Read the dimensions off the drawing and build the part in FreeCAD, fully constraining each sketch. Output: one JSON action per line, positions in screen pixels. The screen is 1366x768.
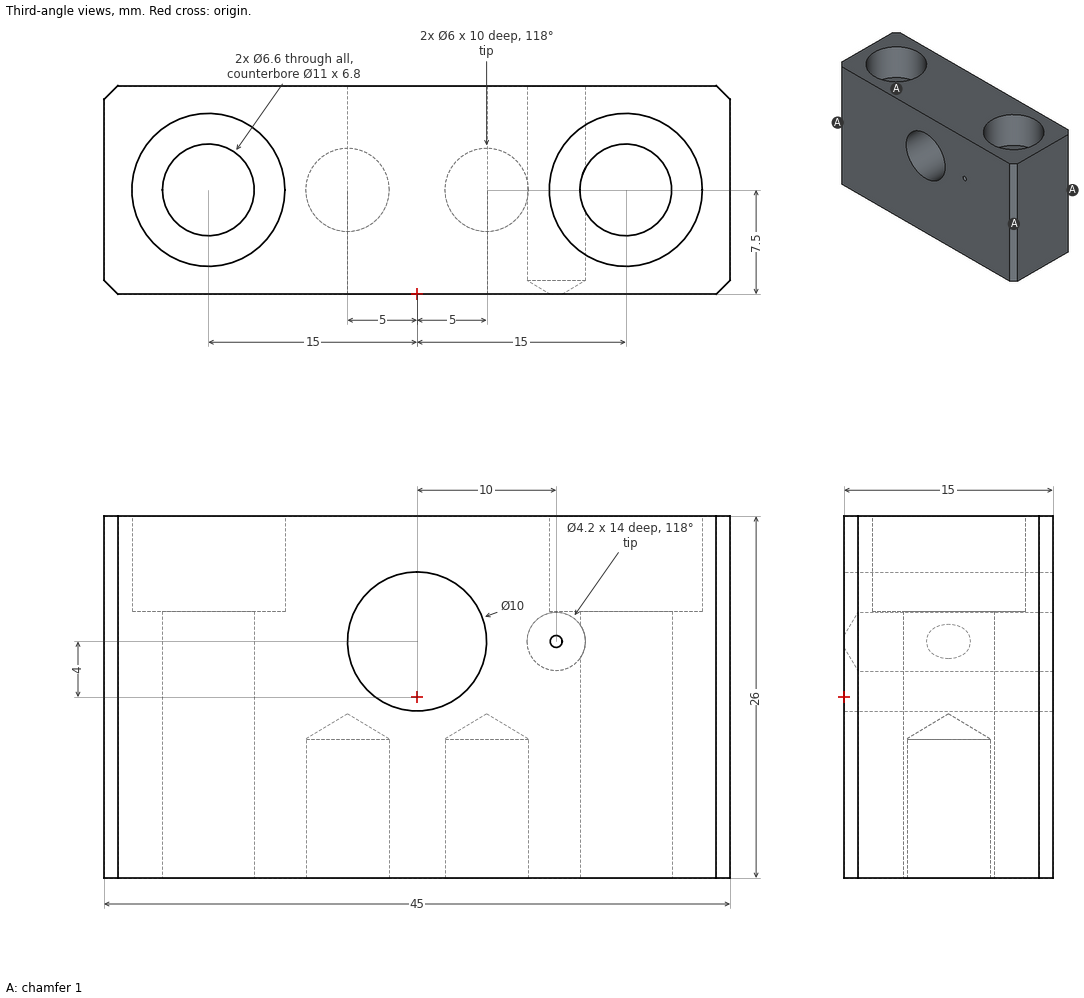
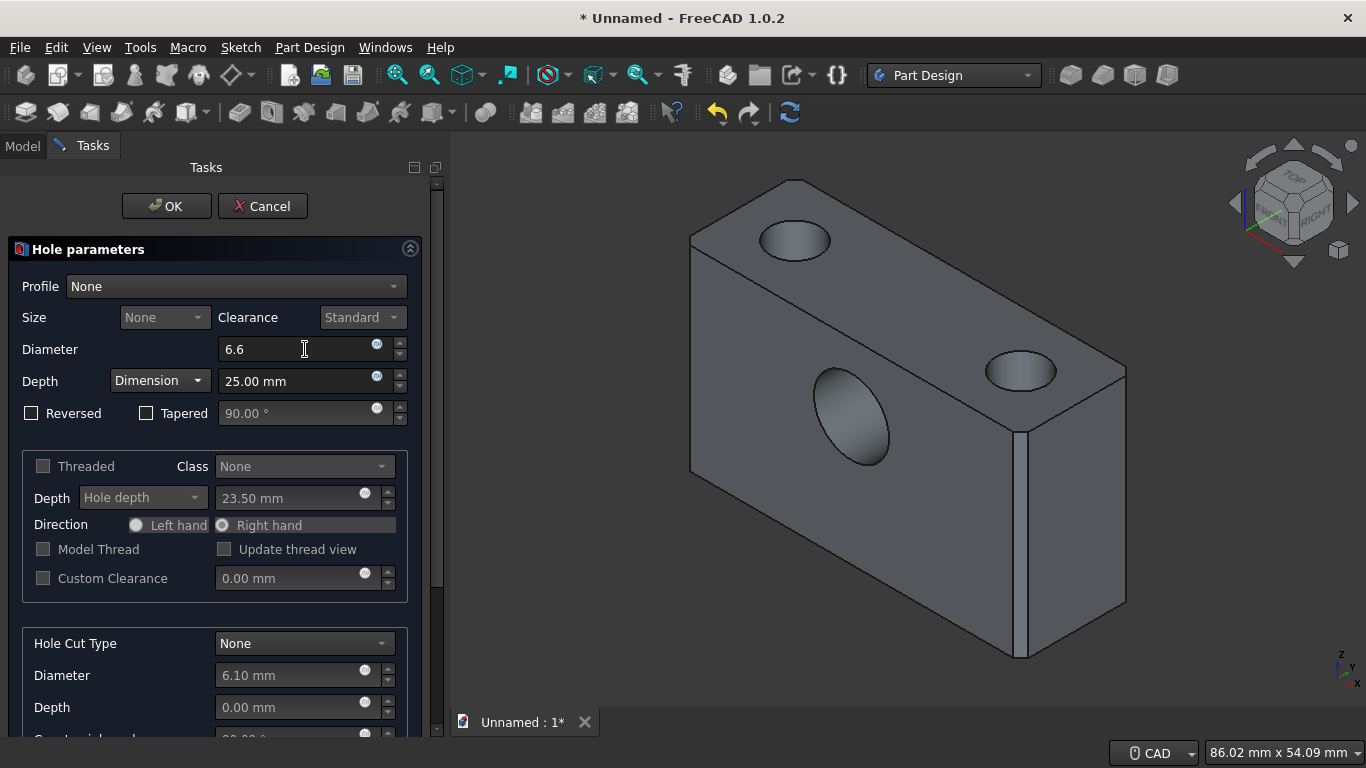
{"action": "left_click", "coordinate": [161, 380]}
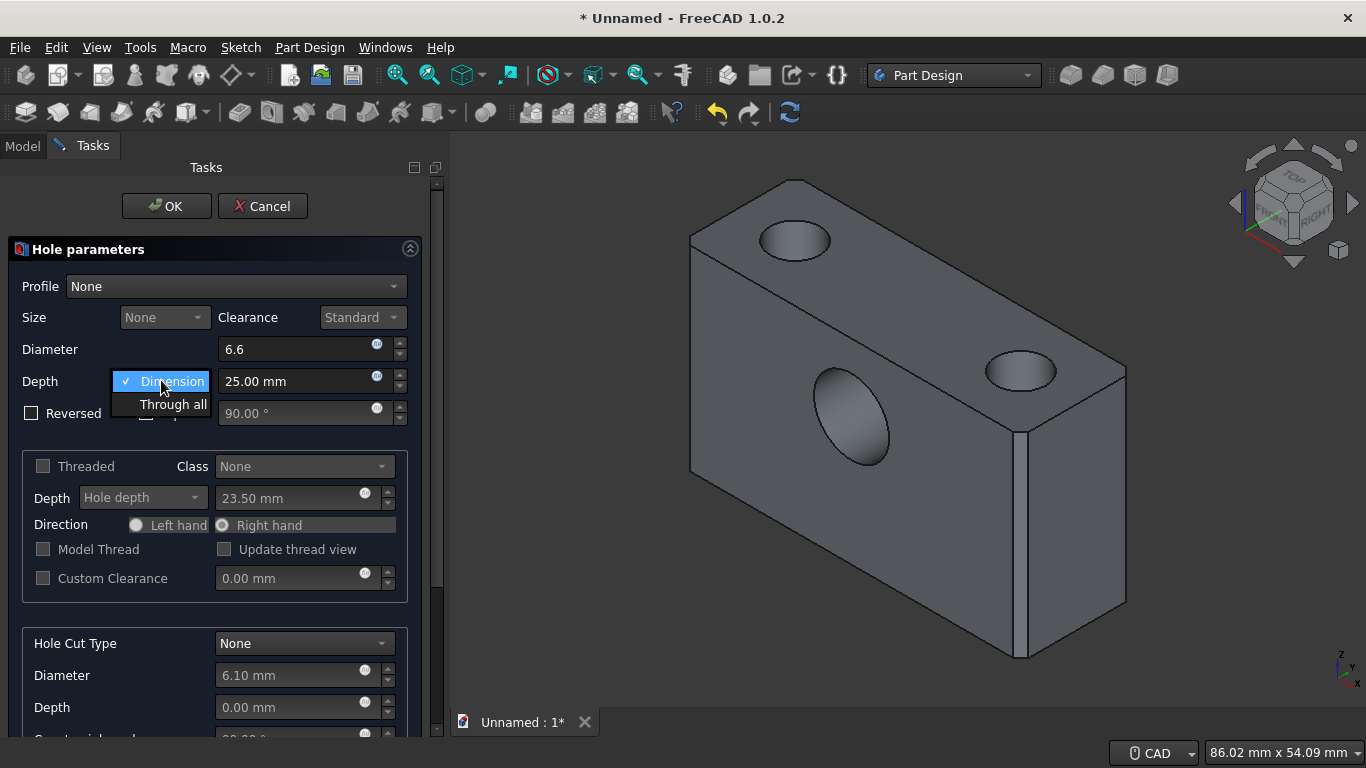
{"action": "left_click", "coordinate": [160, 404]}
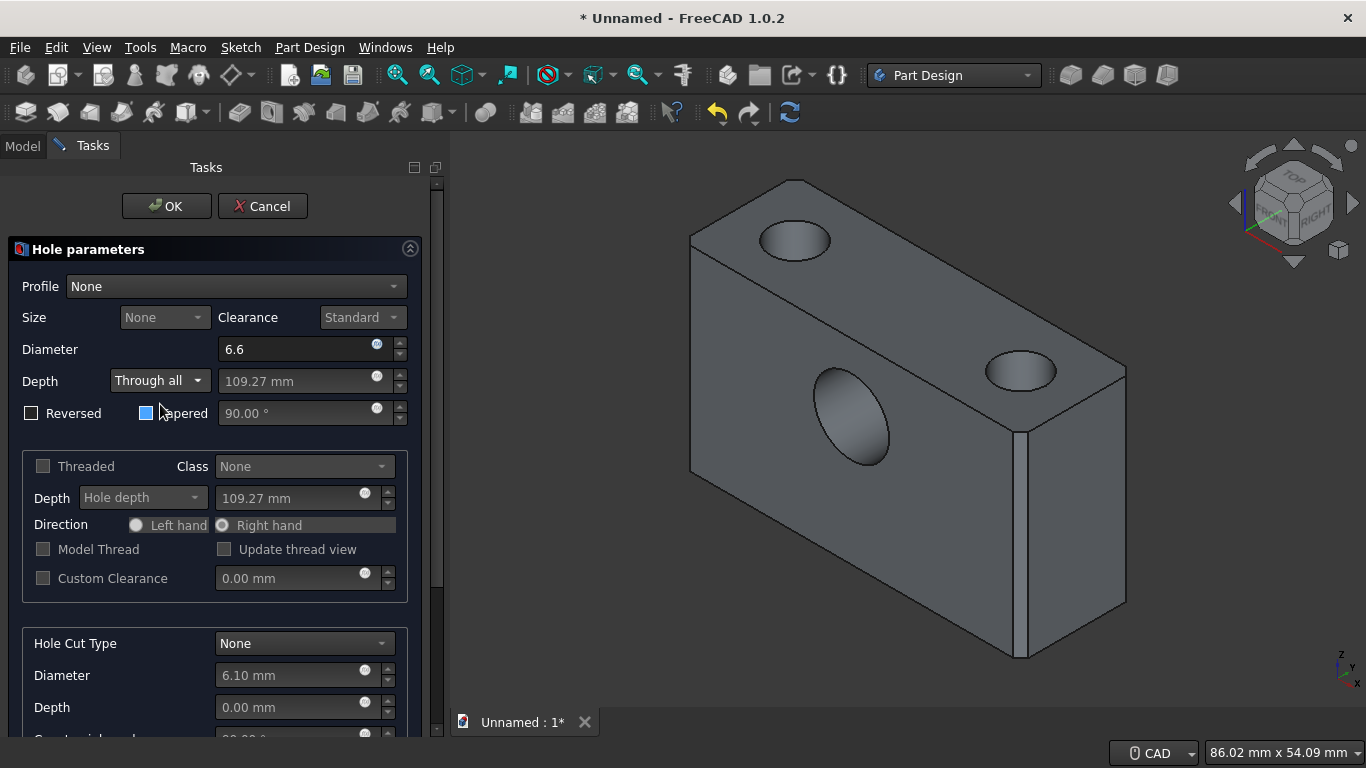
{"action": "left_click", "coordinate": [306, 644]}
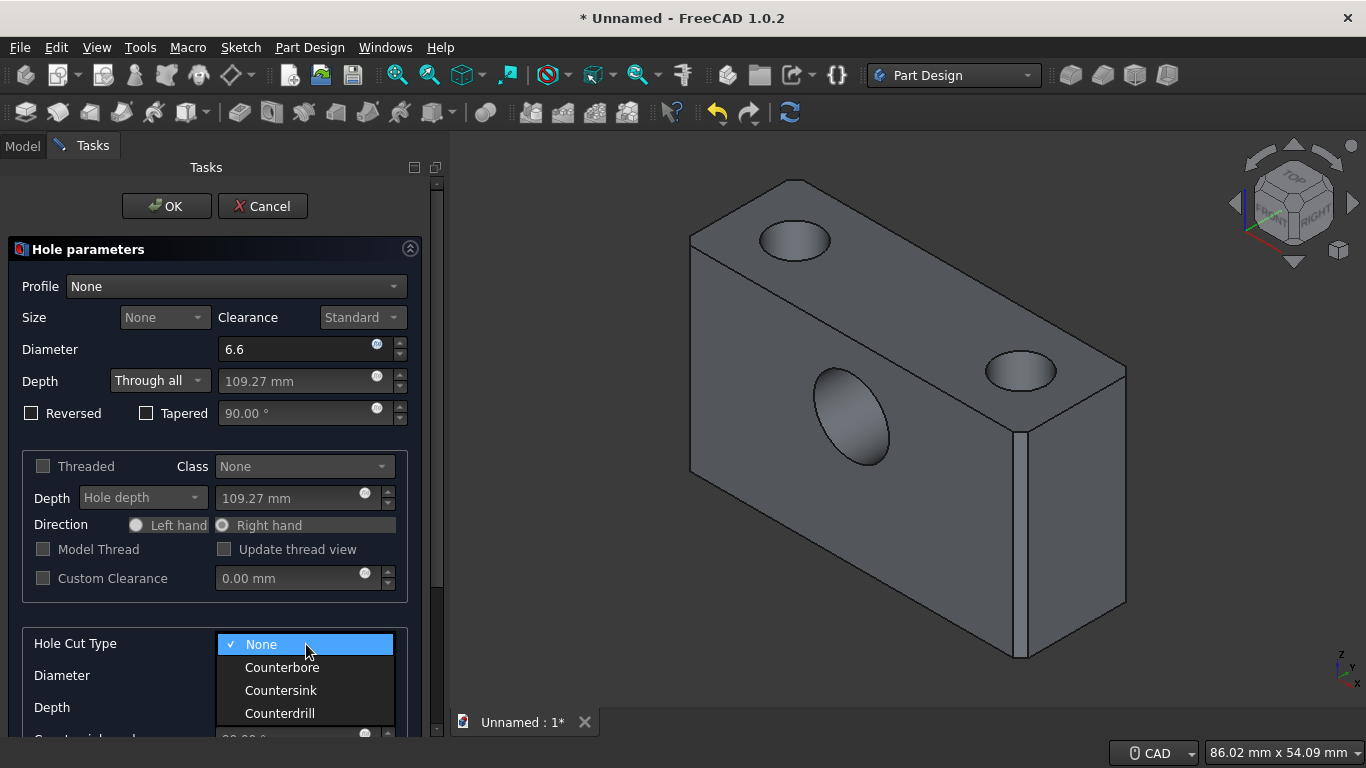
{"action": "left_click", "coordinate": [304, 668]}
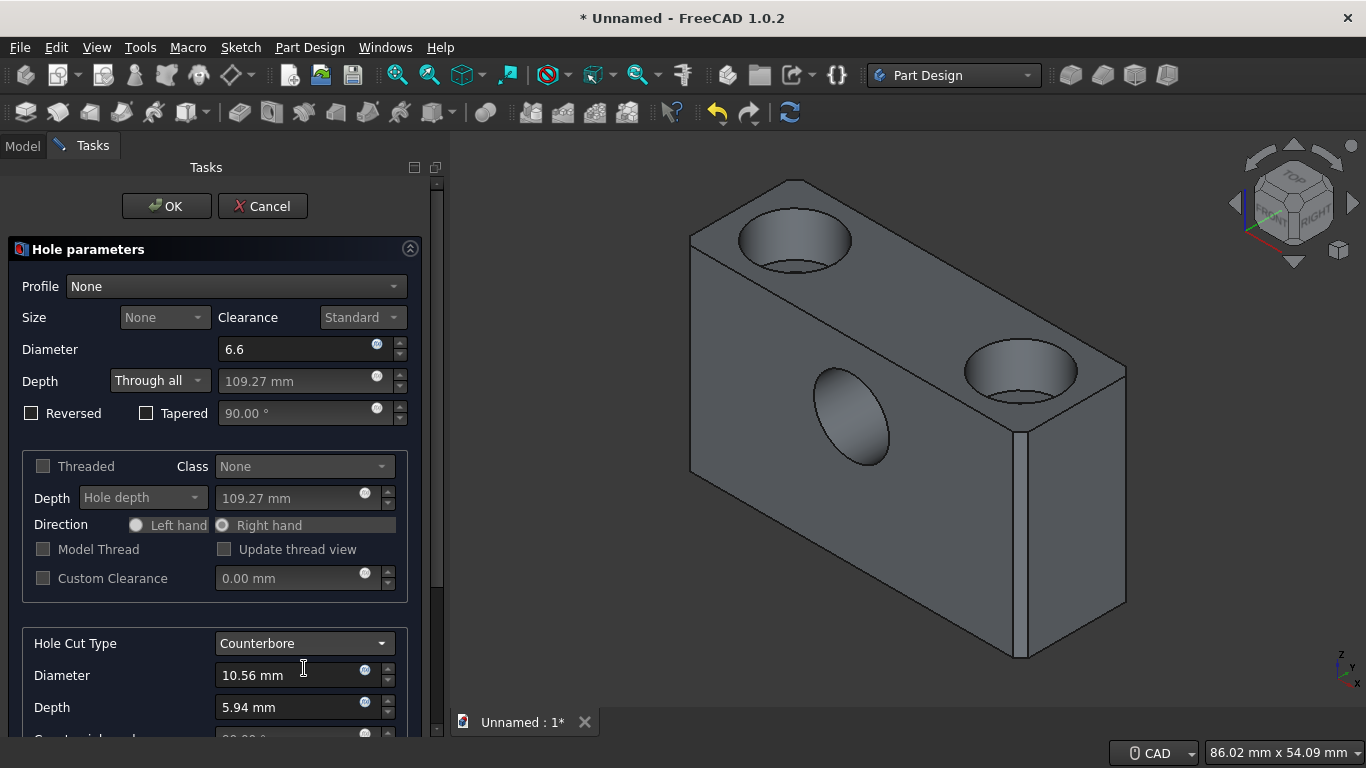
{"action": "triple_click", "coordinate": [298, 675]}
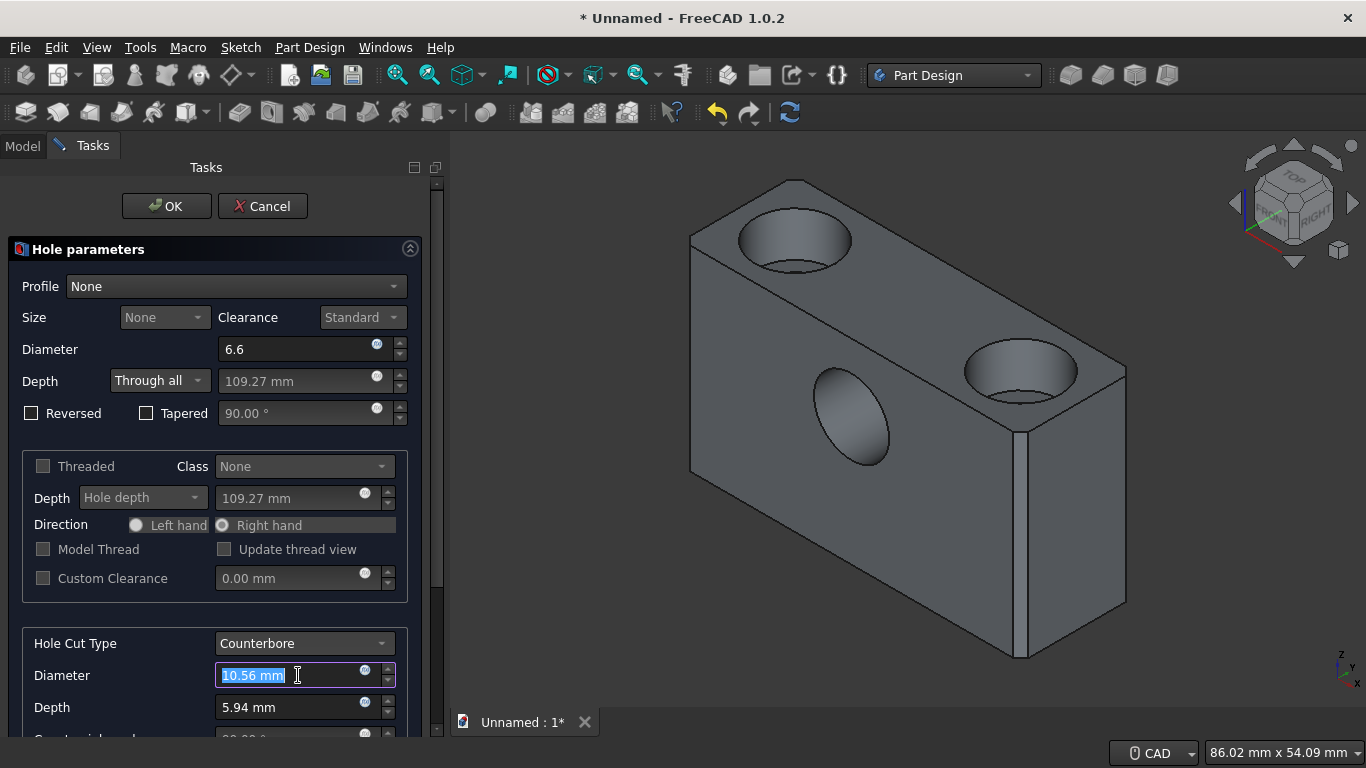
{"action": "type", "text": "11"}
{"action": "key", "text": "Tab"}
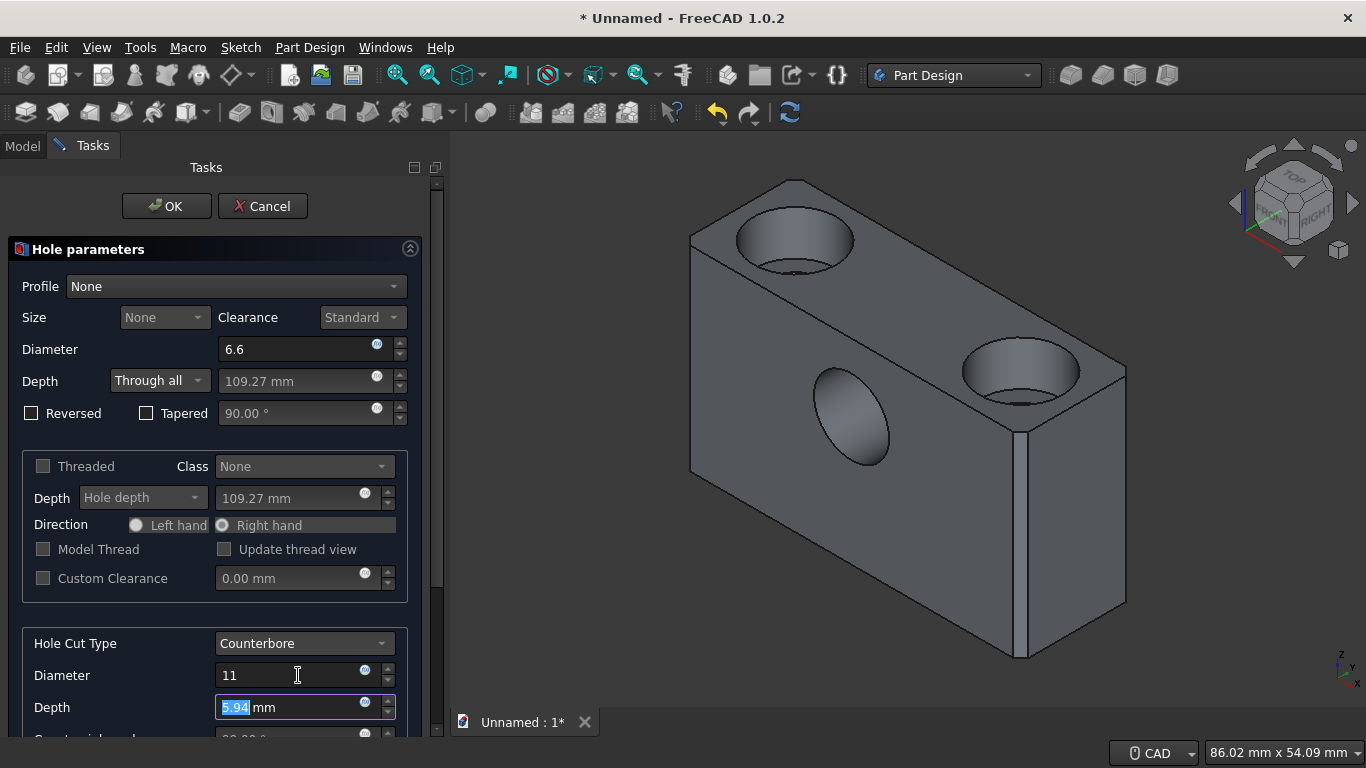
{"action": "type", "text": "6.8"}
{"action": "key", "text": "Tab"}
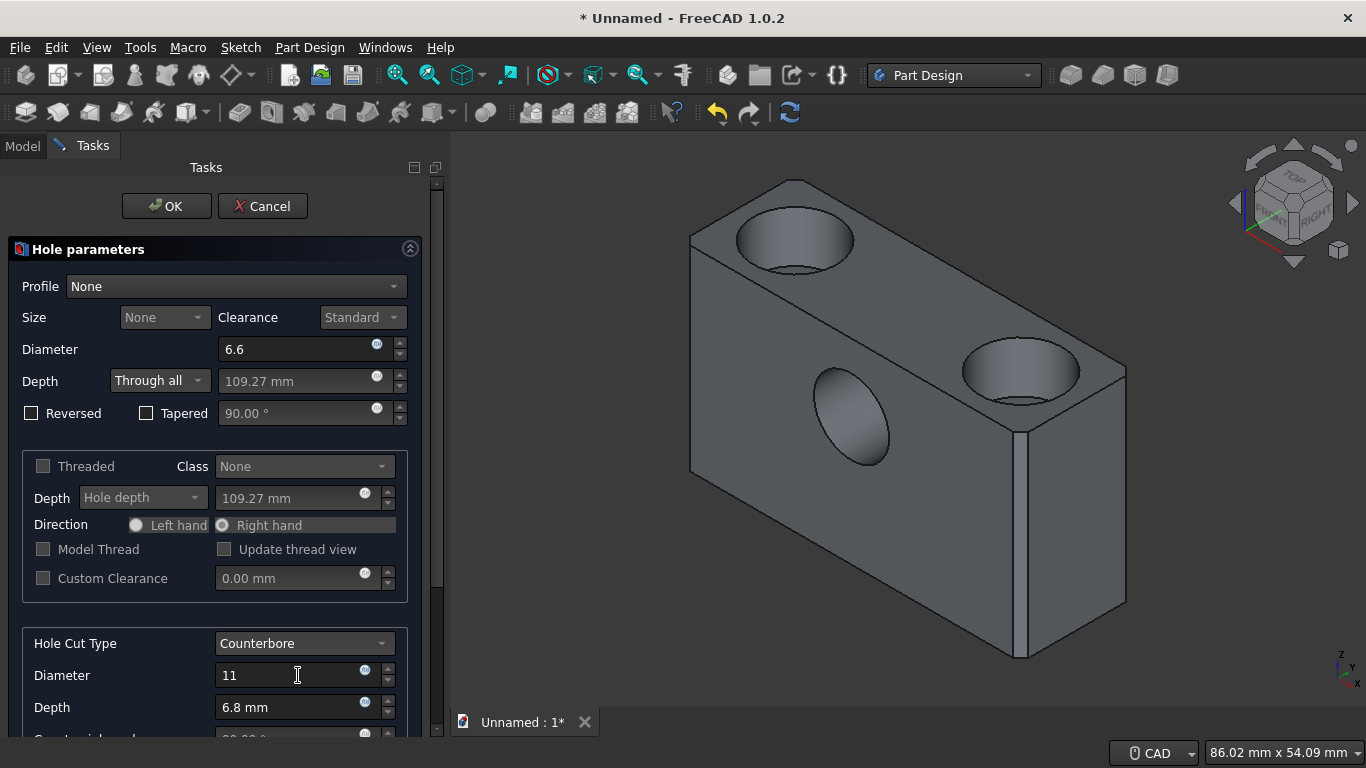
{"action": "left_click", "coordinate": [167, 206]}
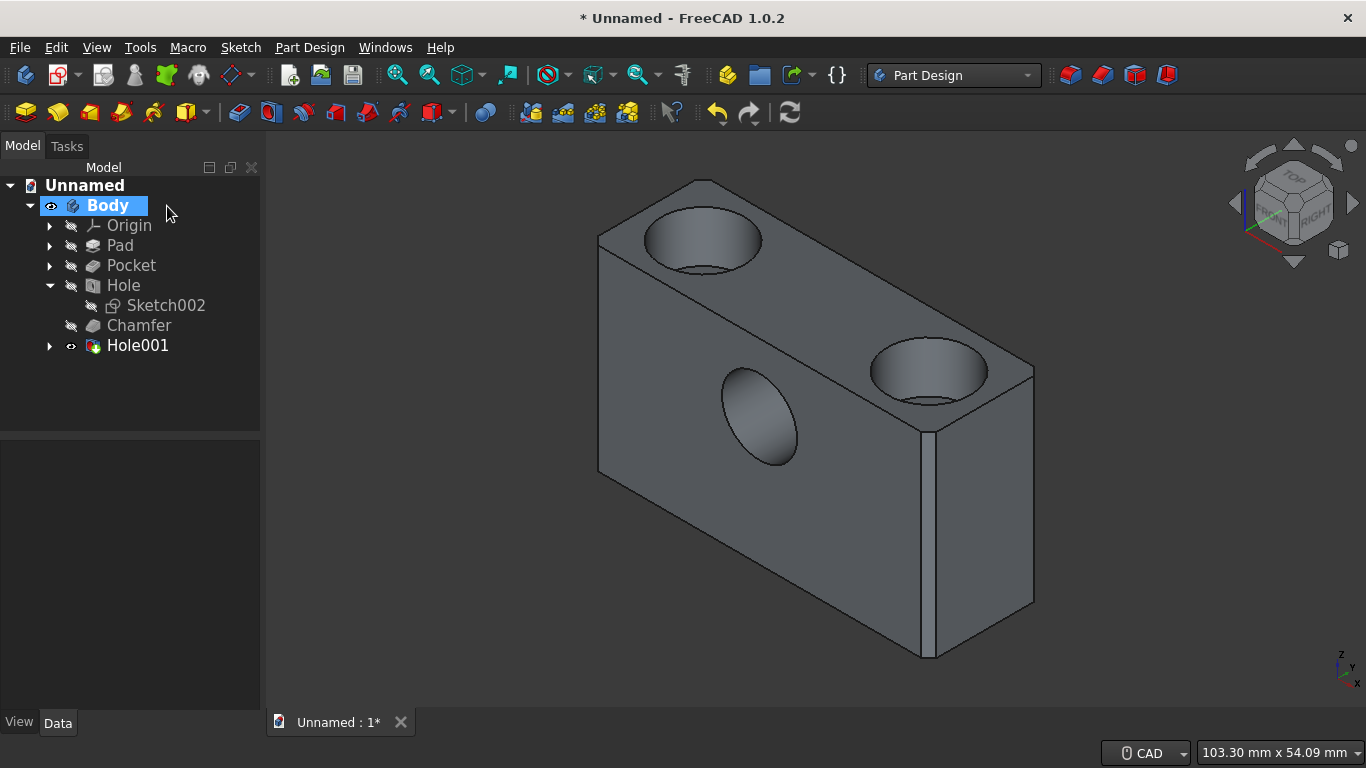
{"action": "key", "text": "4"}